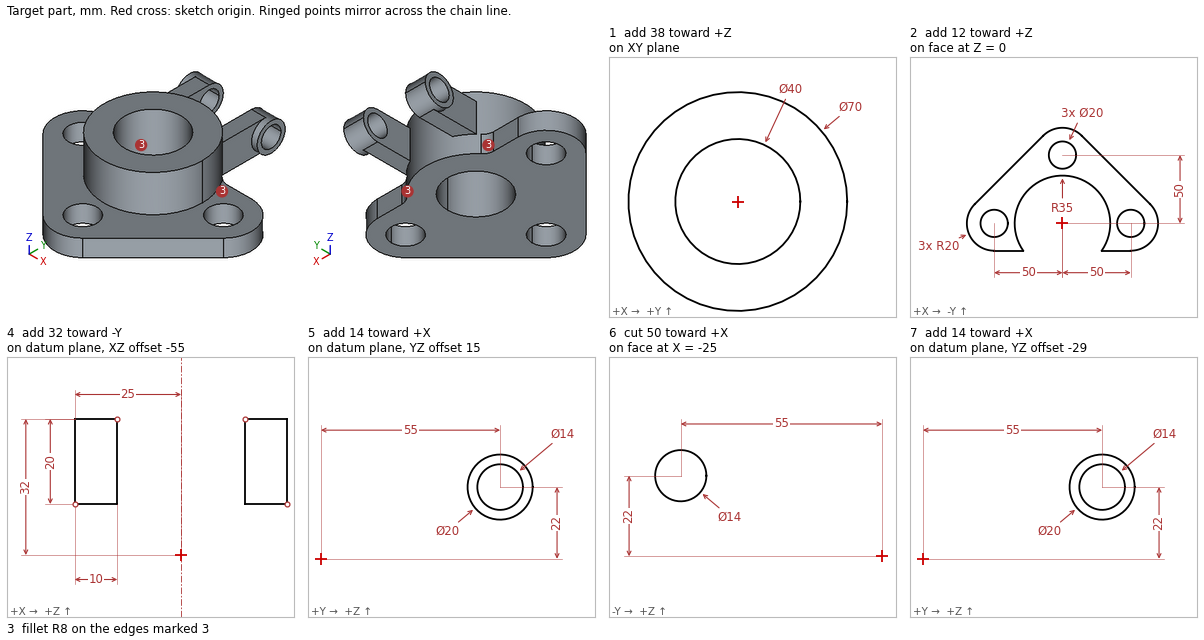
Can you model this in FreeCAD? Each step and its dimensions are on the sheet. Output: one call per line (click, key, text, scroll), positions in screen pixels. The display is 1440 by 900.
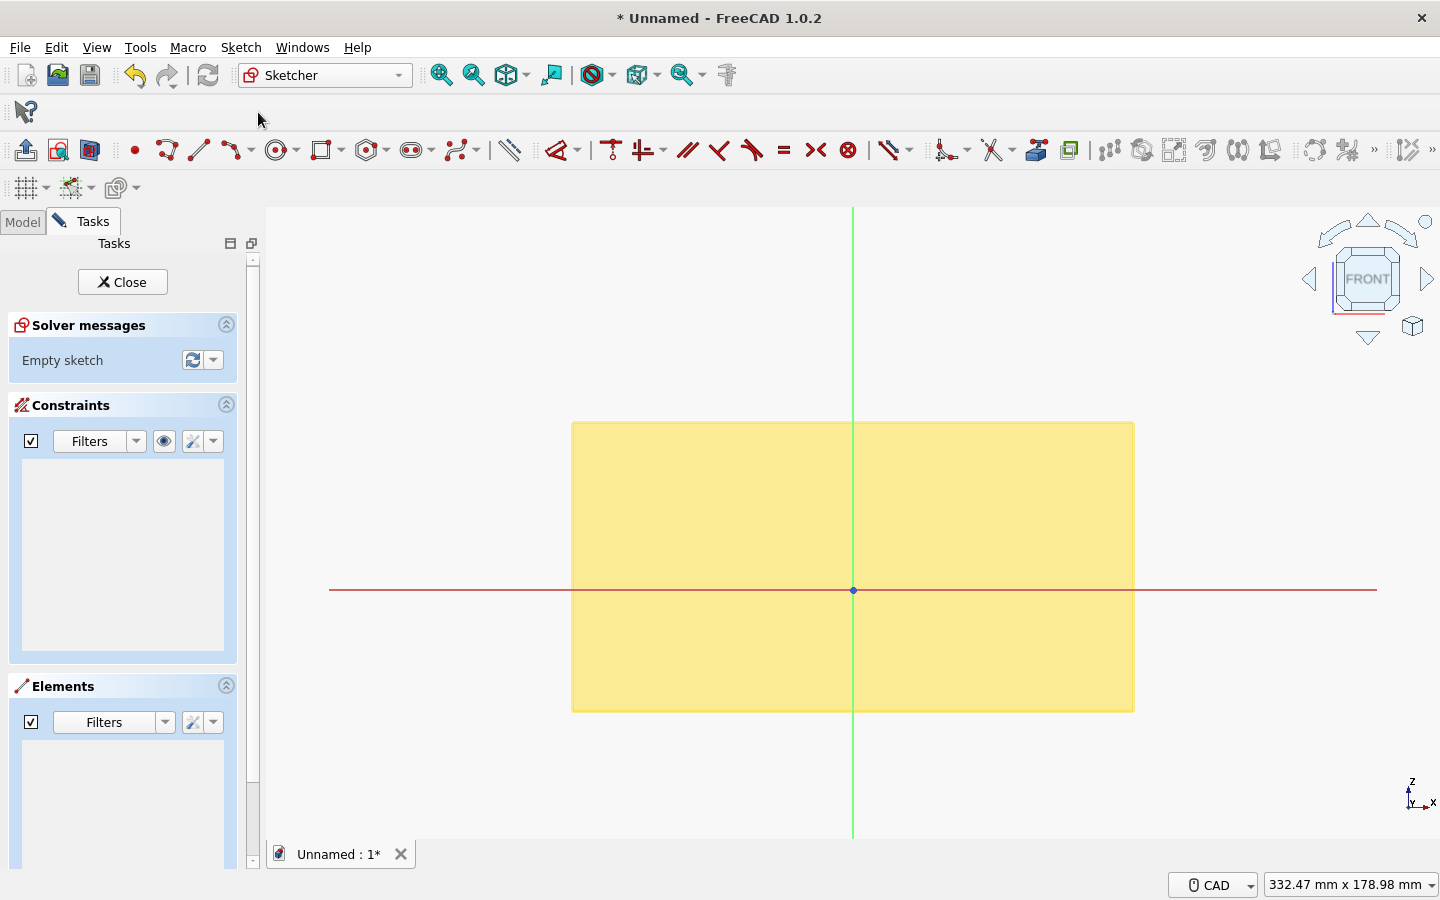
scroll(883, 538, up, 6)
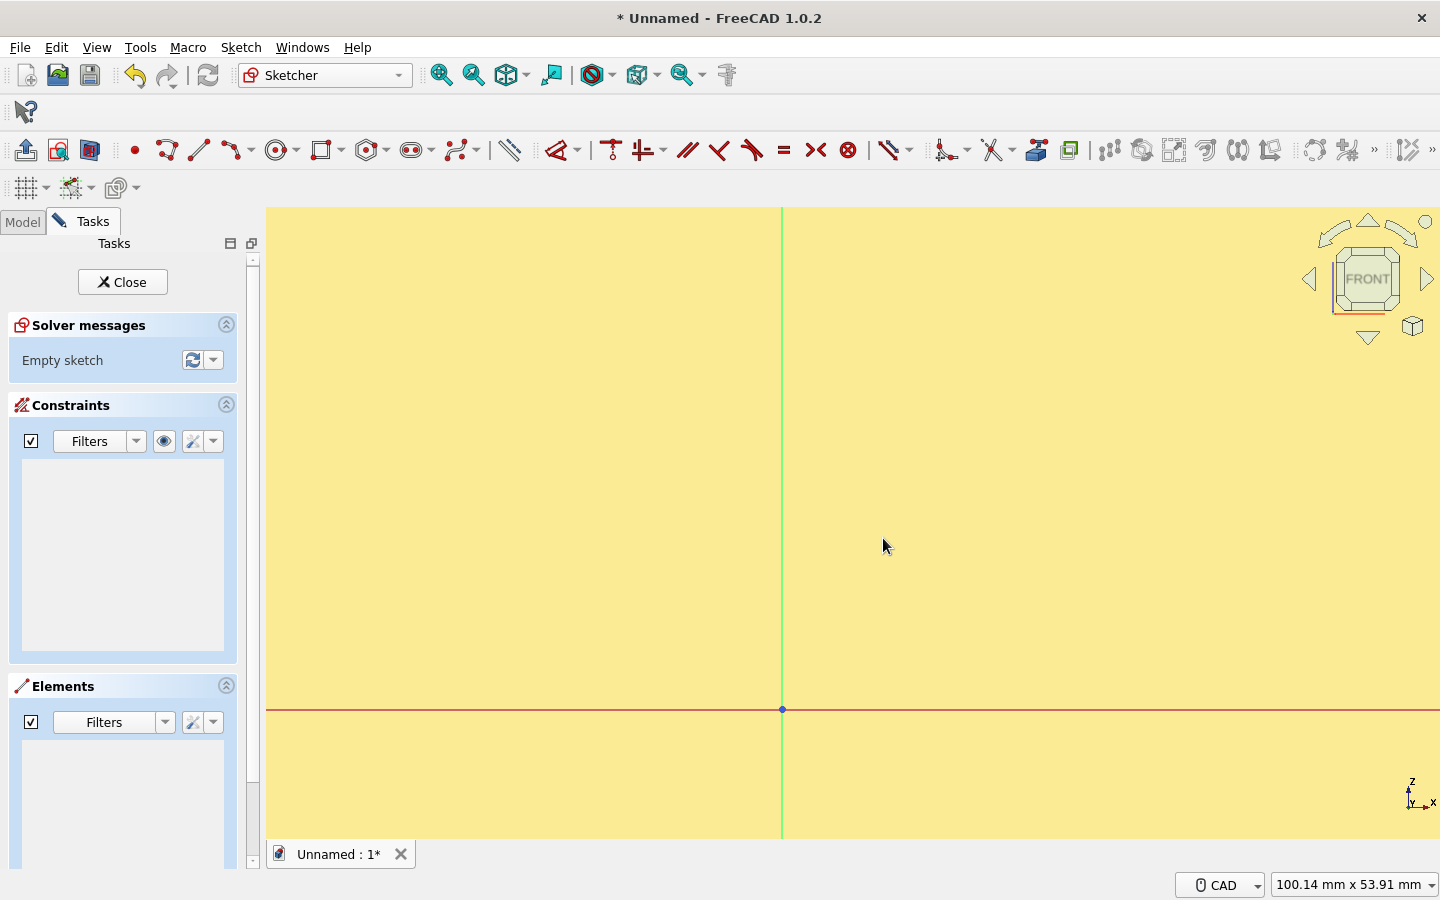
key(g)
key(r)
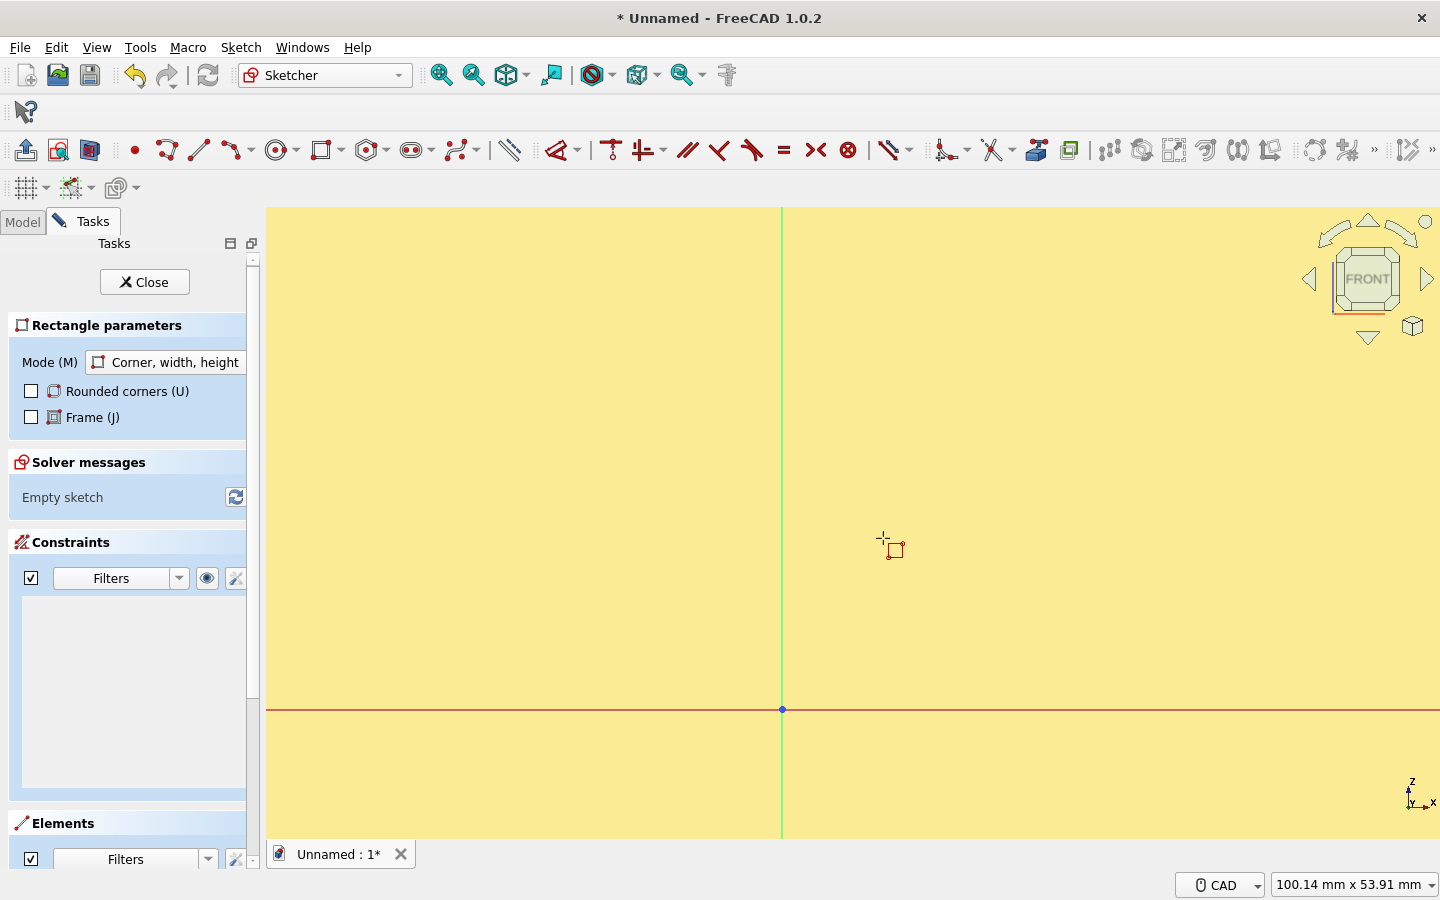
click(489, 335)
click(606, 569)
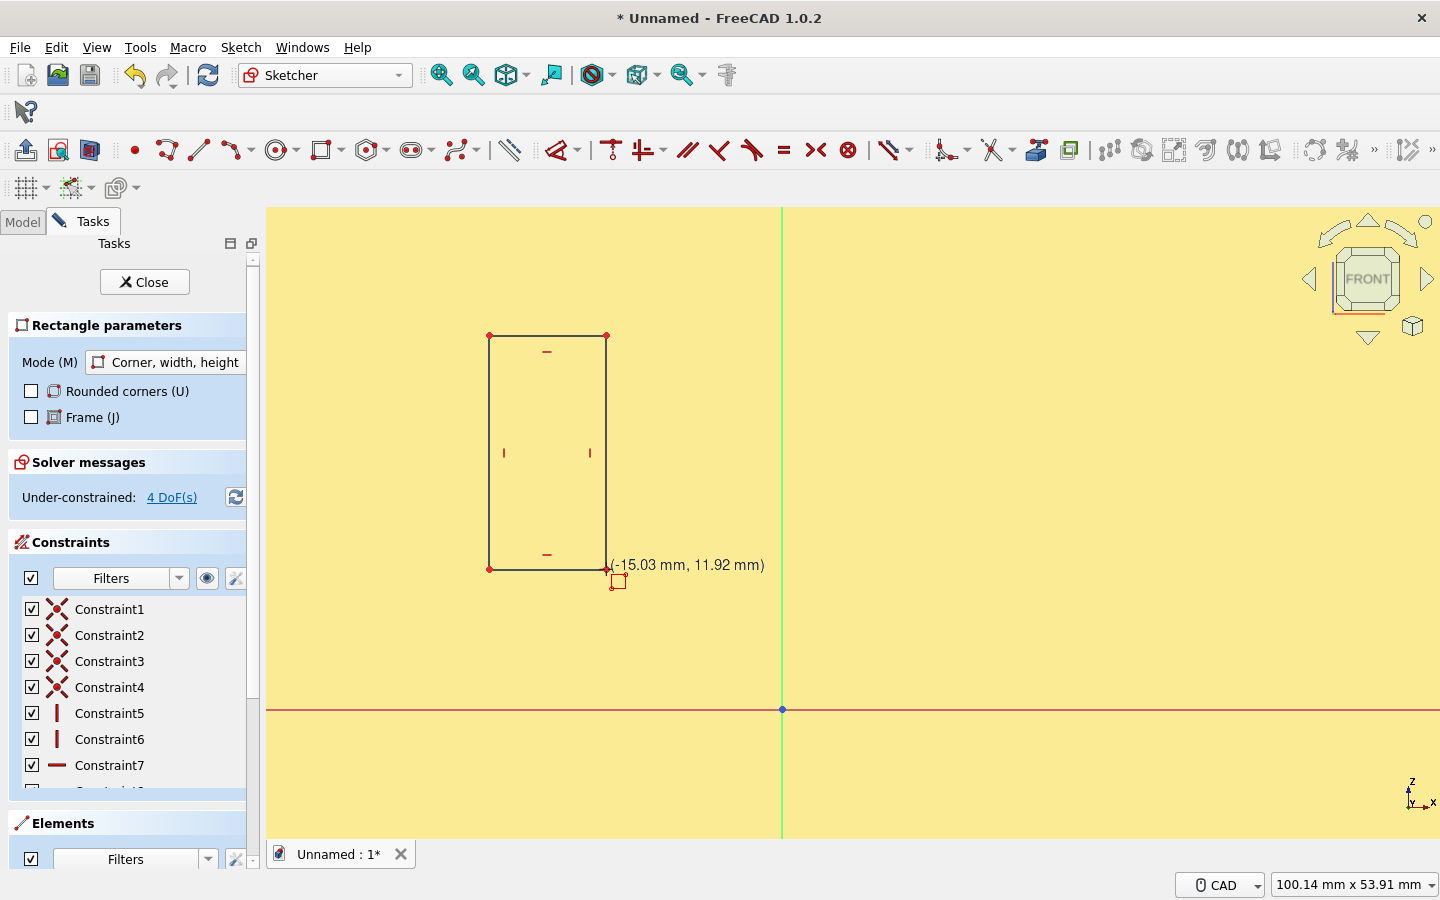
click(958, 335)
click(1075, 569)
key(Escape)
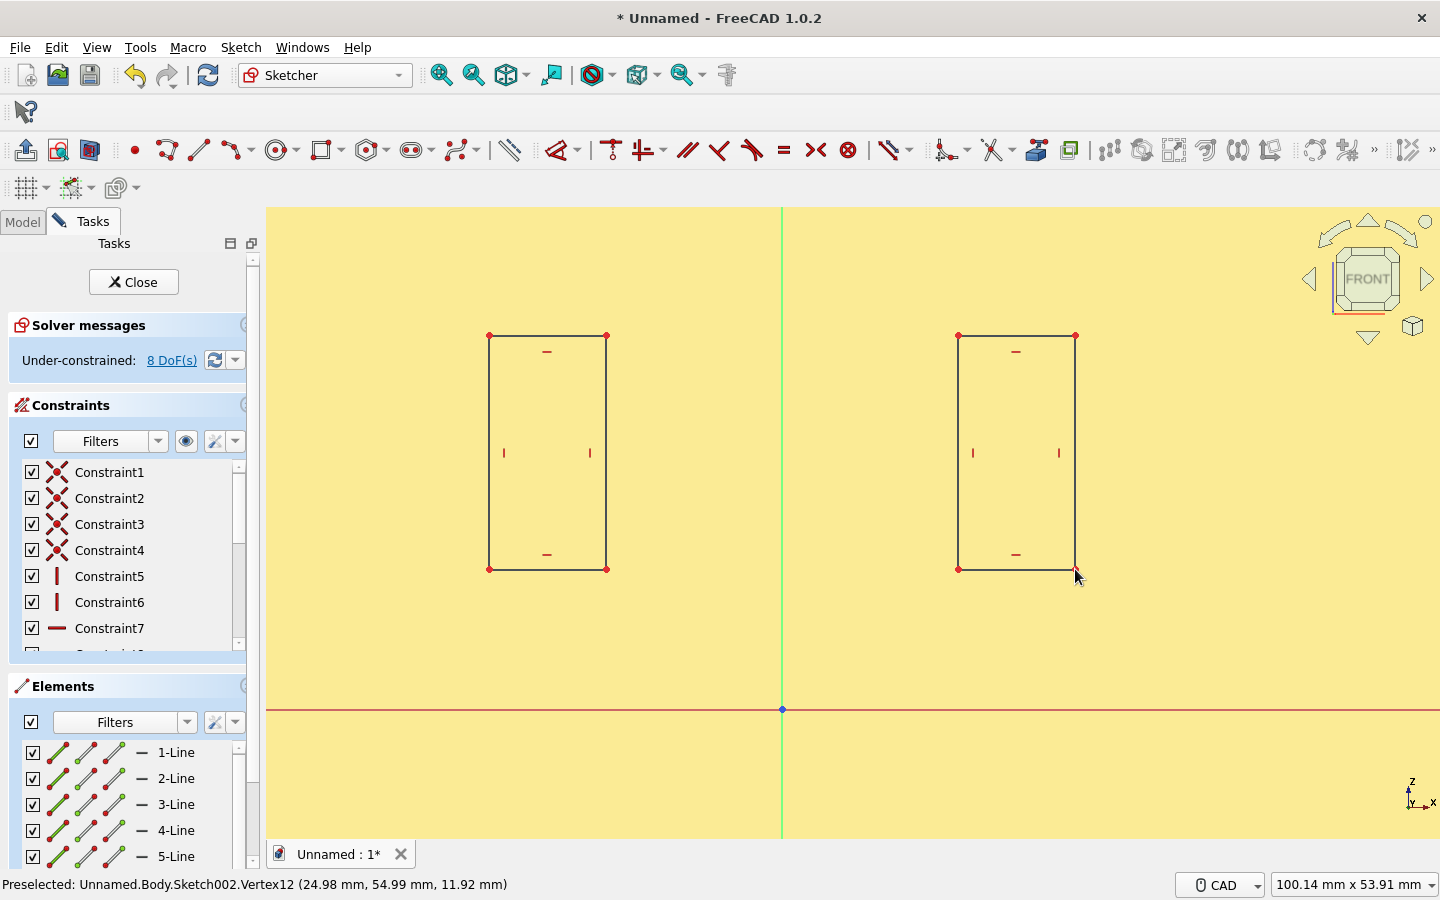
click(606, 336)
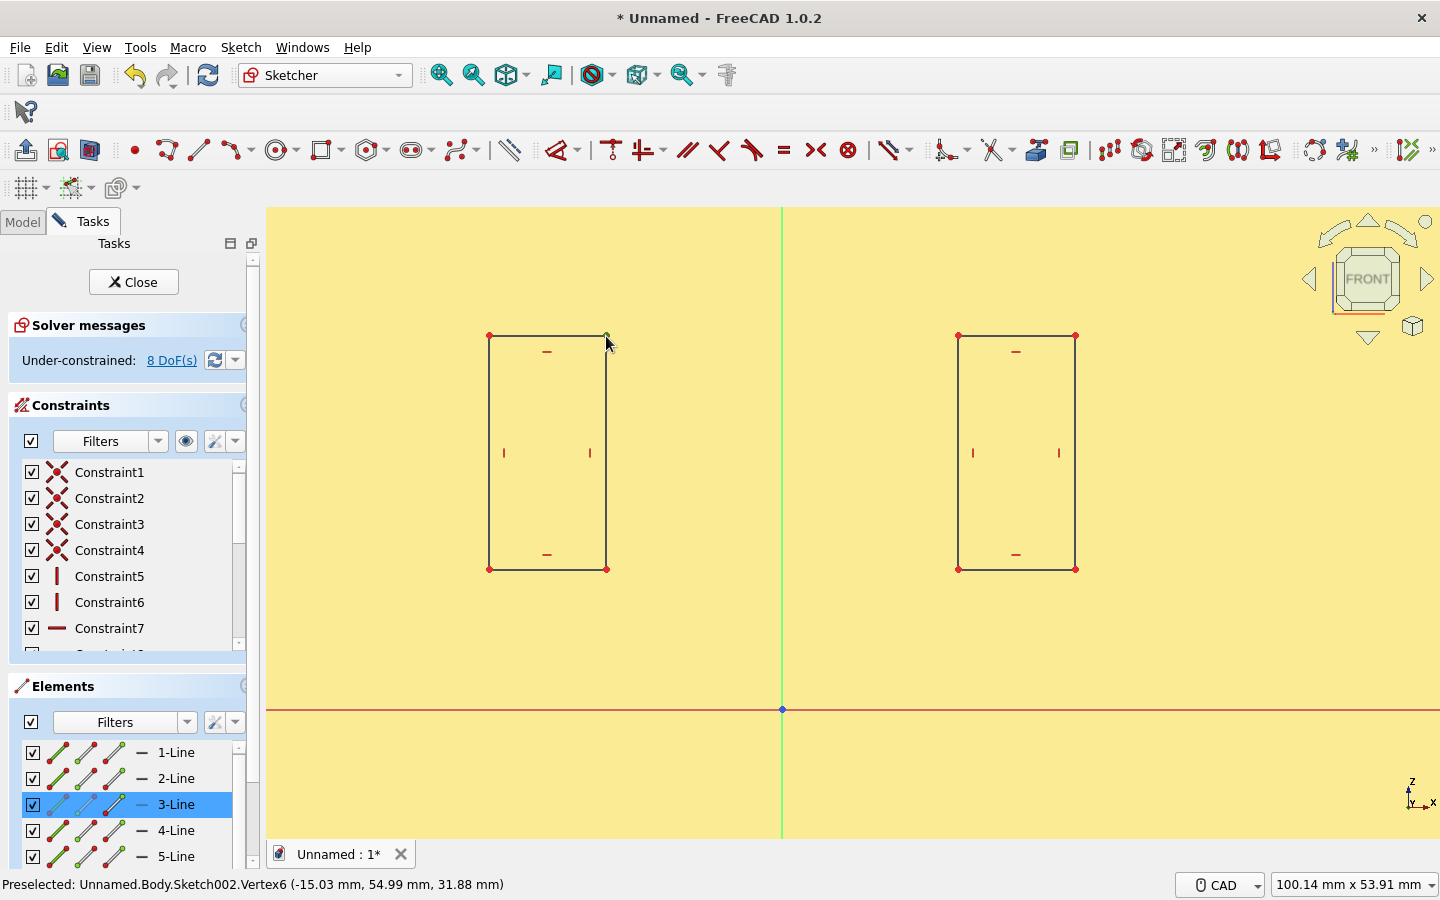
click(958, 336)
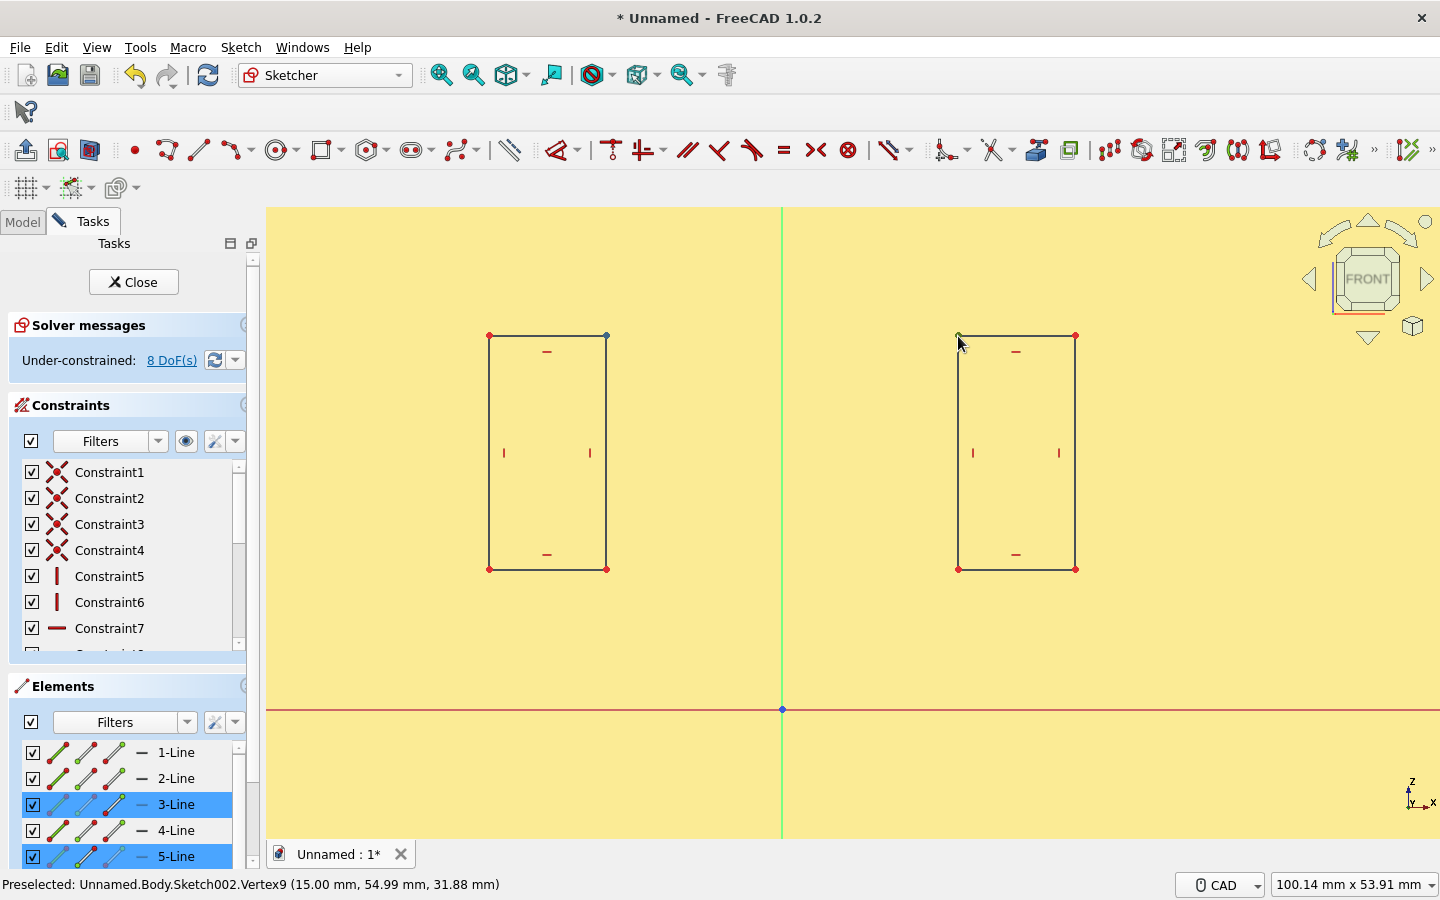
click(782, 770)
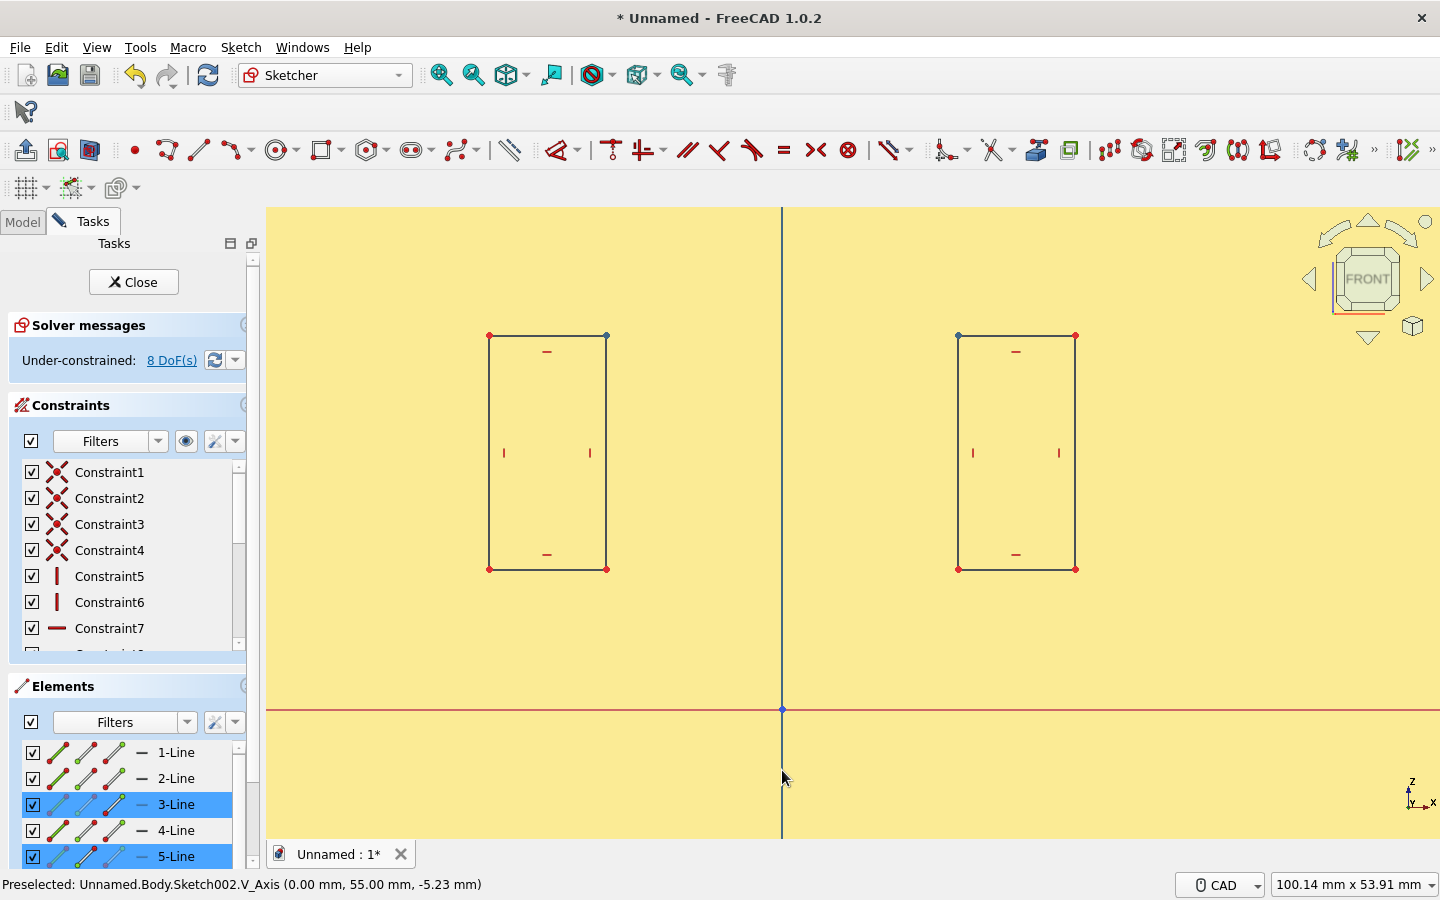
click(816, 150)